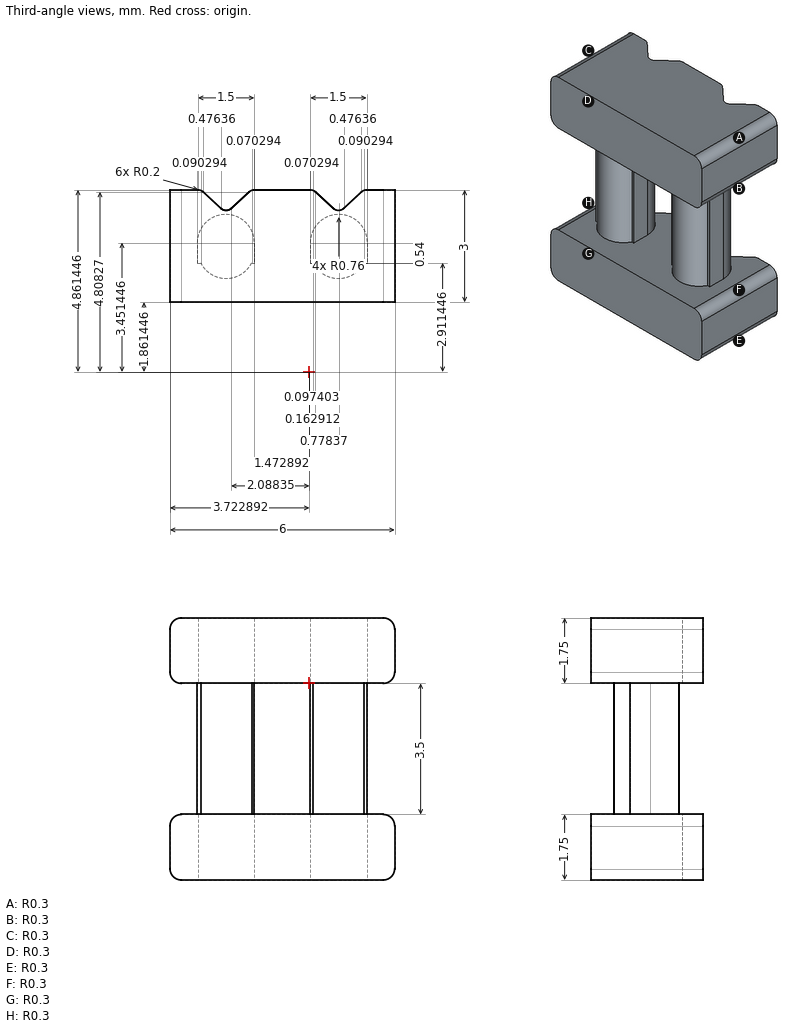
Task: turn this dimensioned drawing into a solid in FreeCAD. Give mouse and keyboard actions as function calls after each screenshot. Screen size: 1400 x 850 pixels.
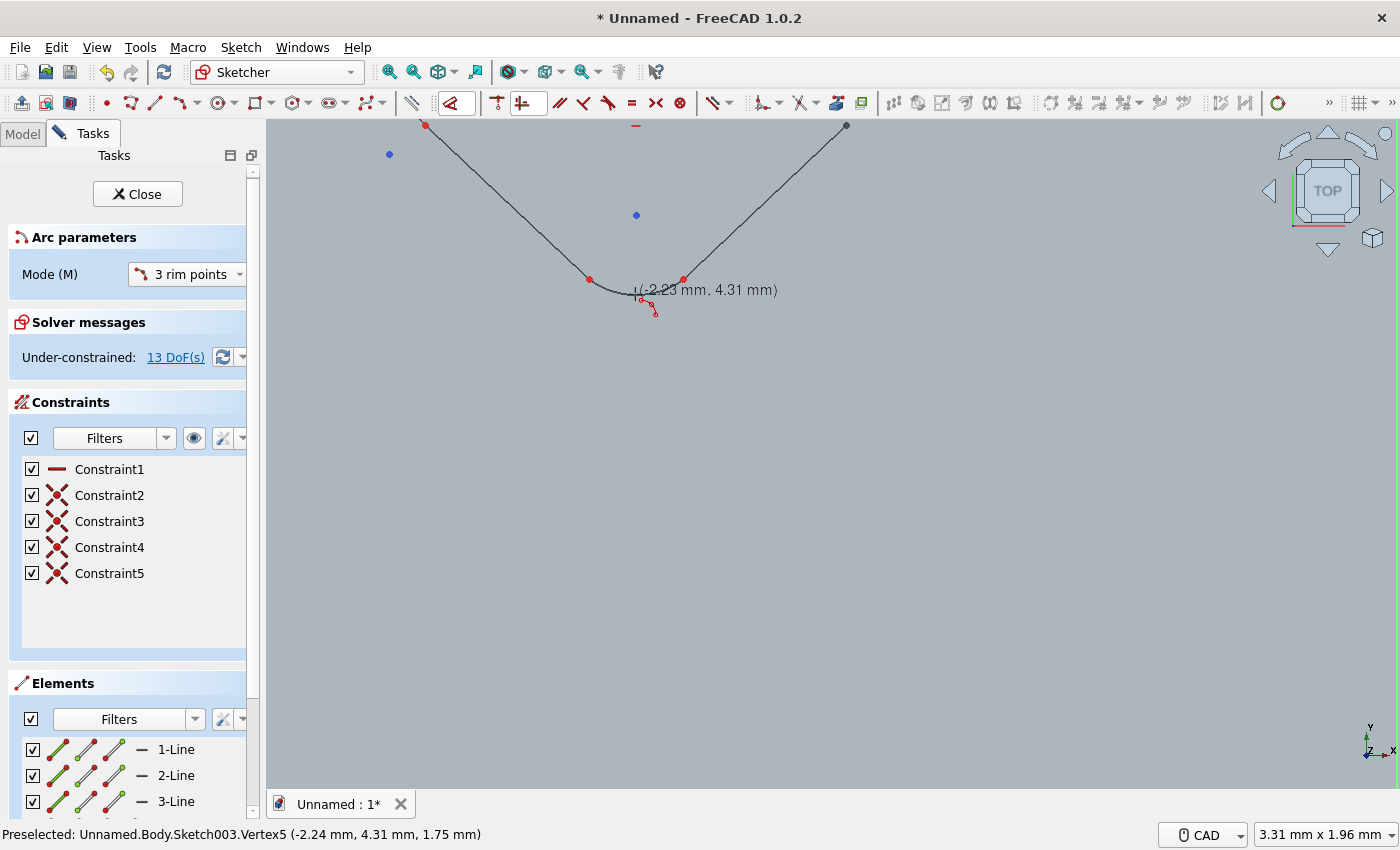
scroll(639, 296, down, 7)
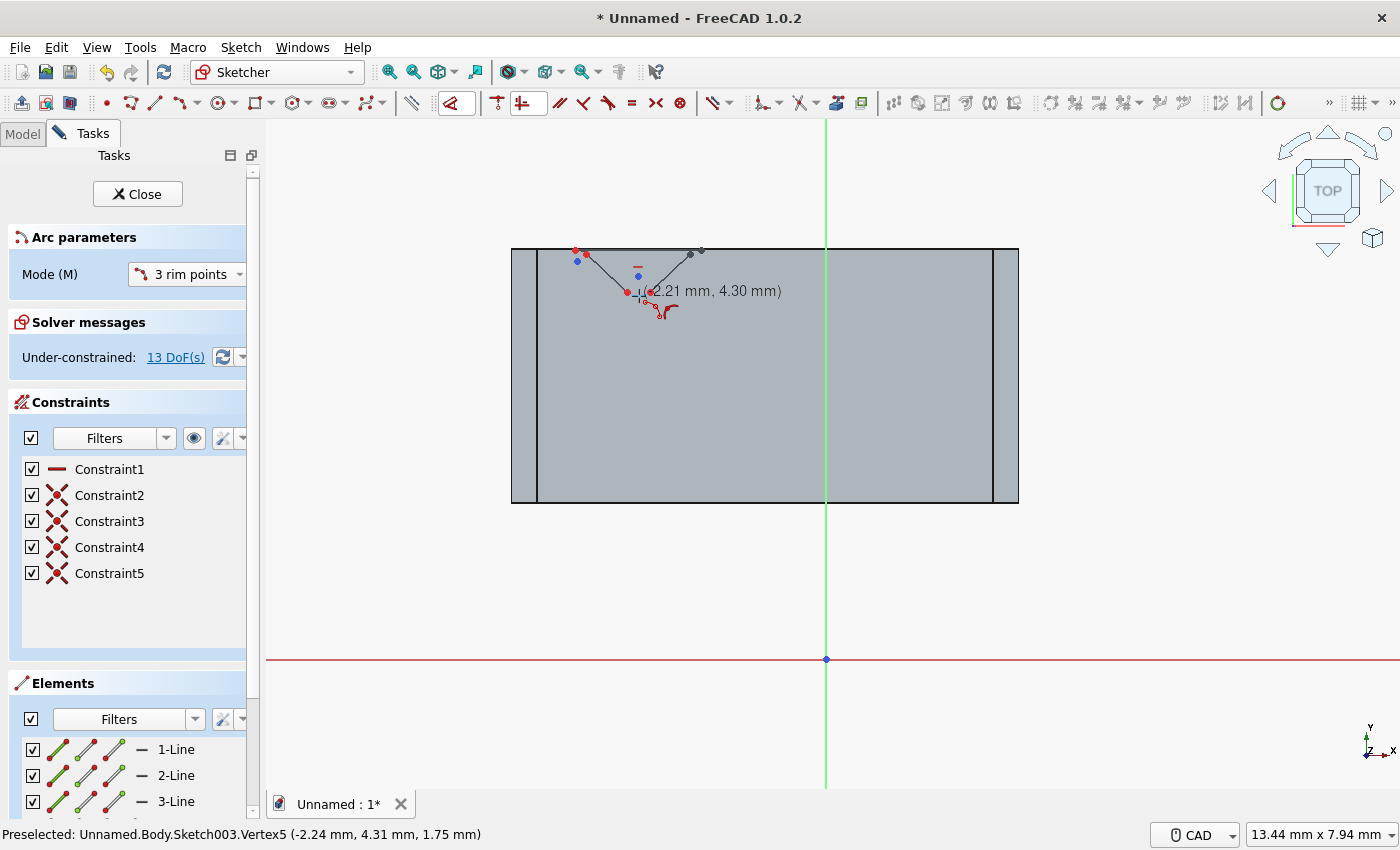
scroll(690, 254, up, 7)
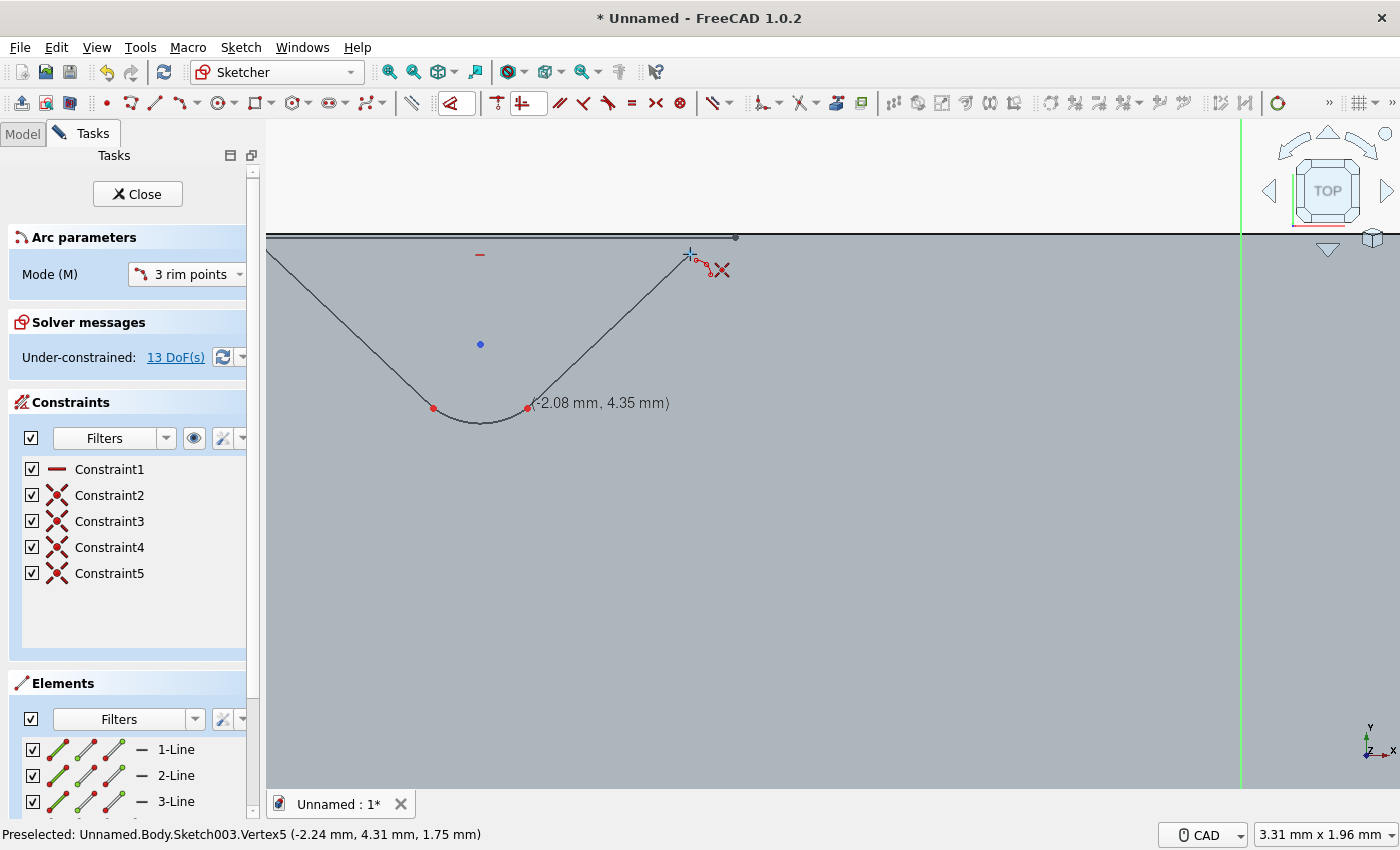
click(690, 254)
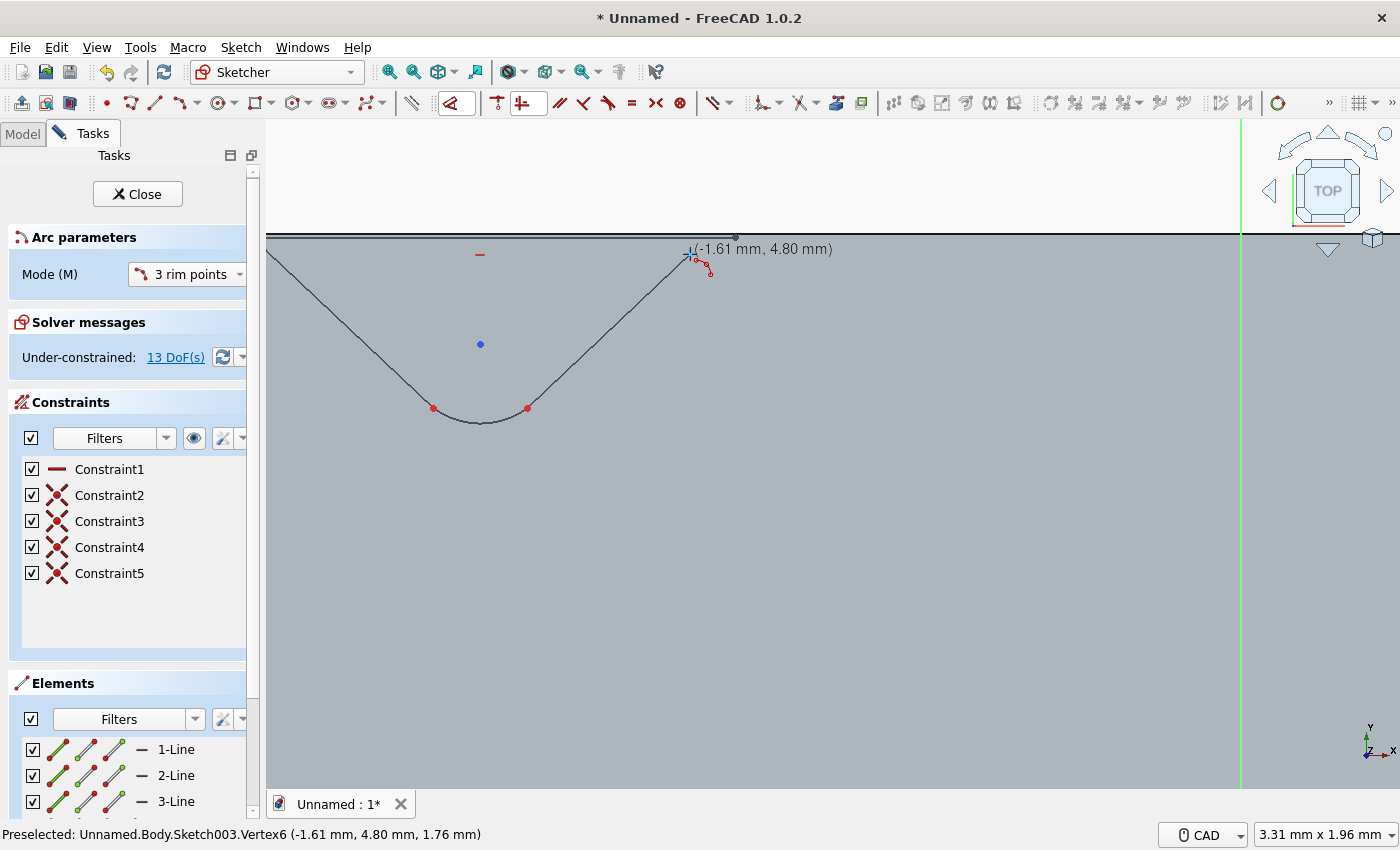
scroll(690, 254, down, 7)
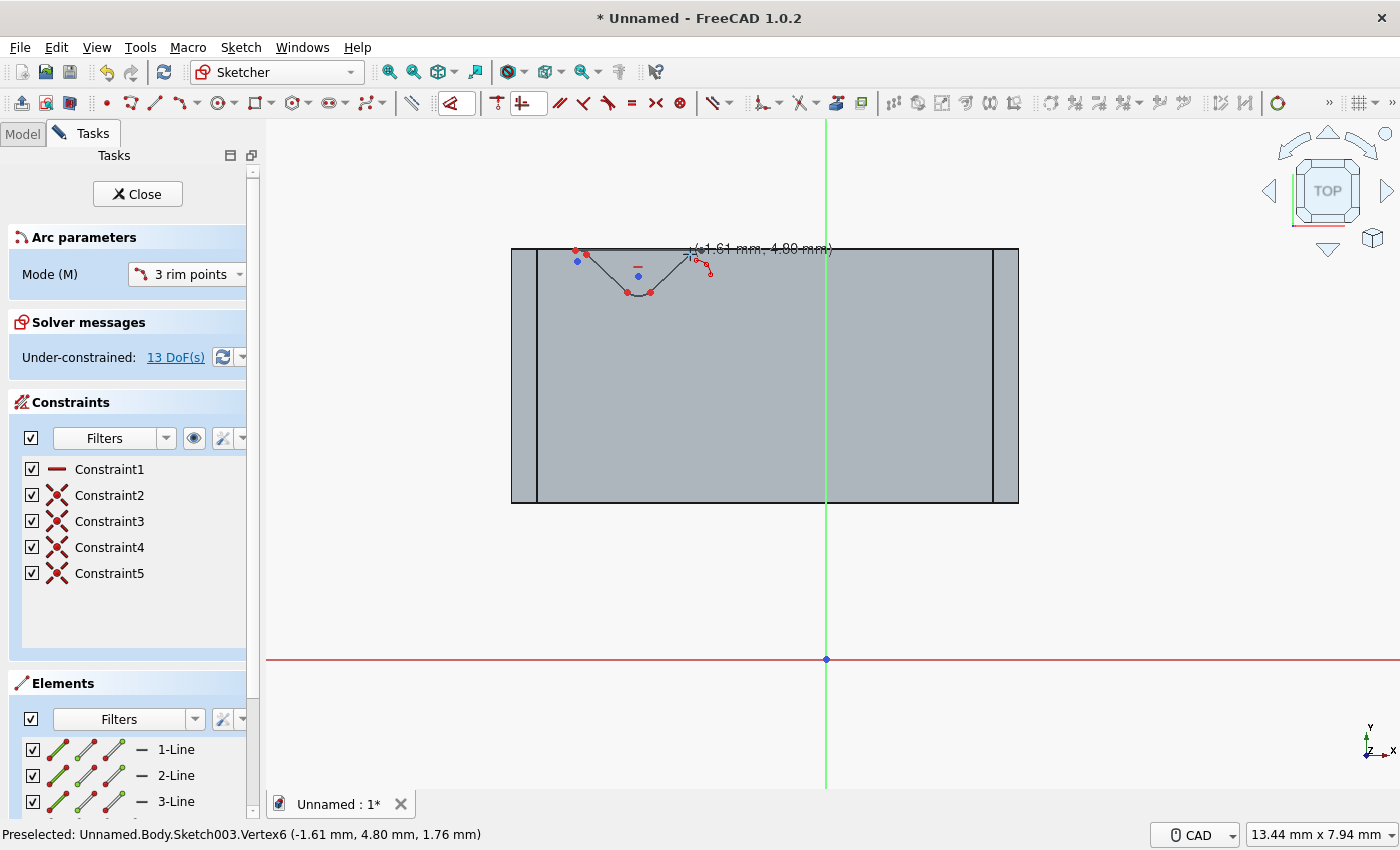
scroll(702, 249, up, 2)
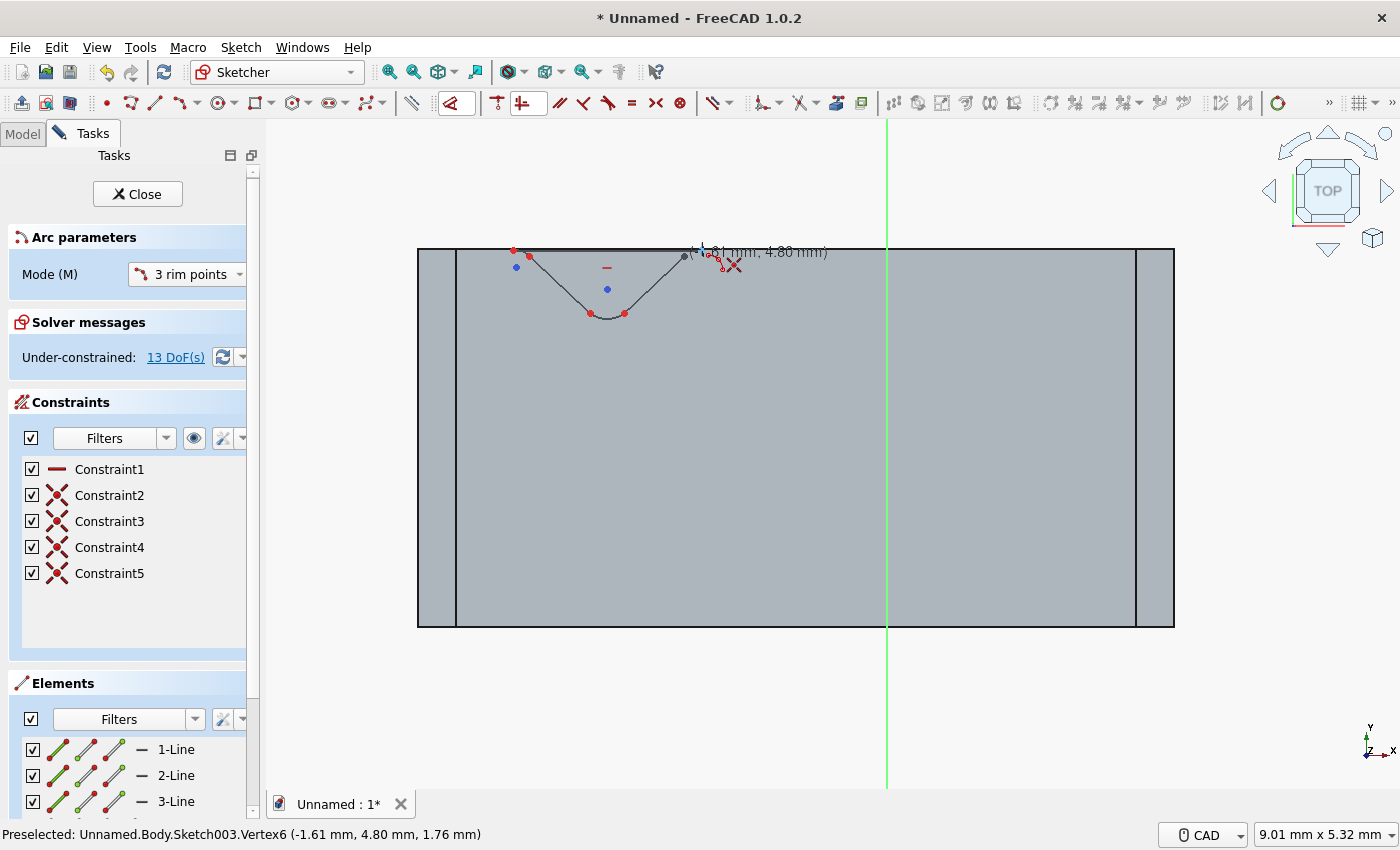
click(701, 251)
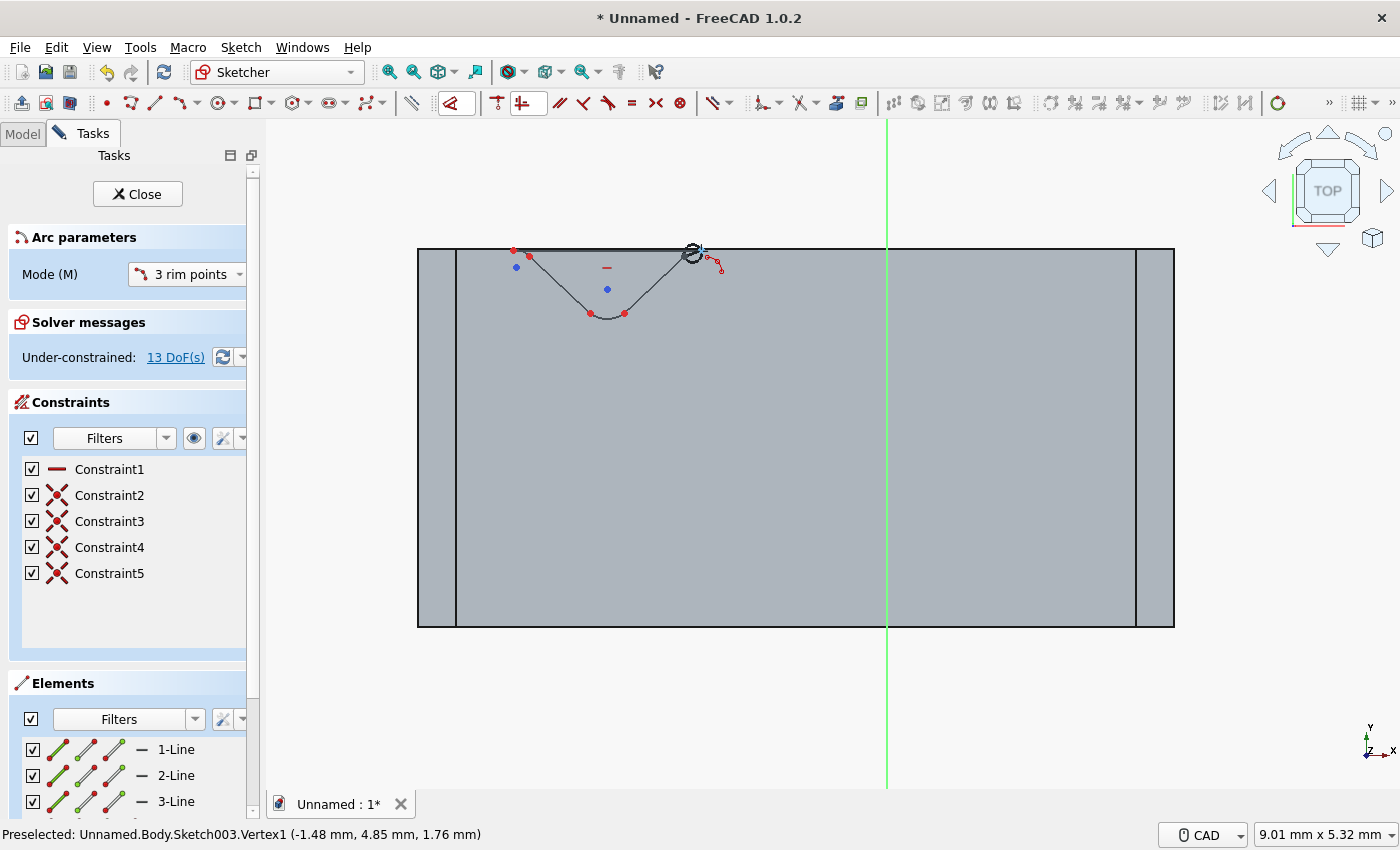
scroll(692, 251, up, 12)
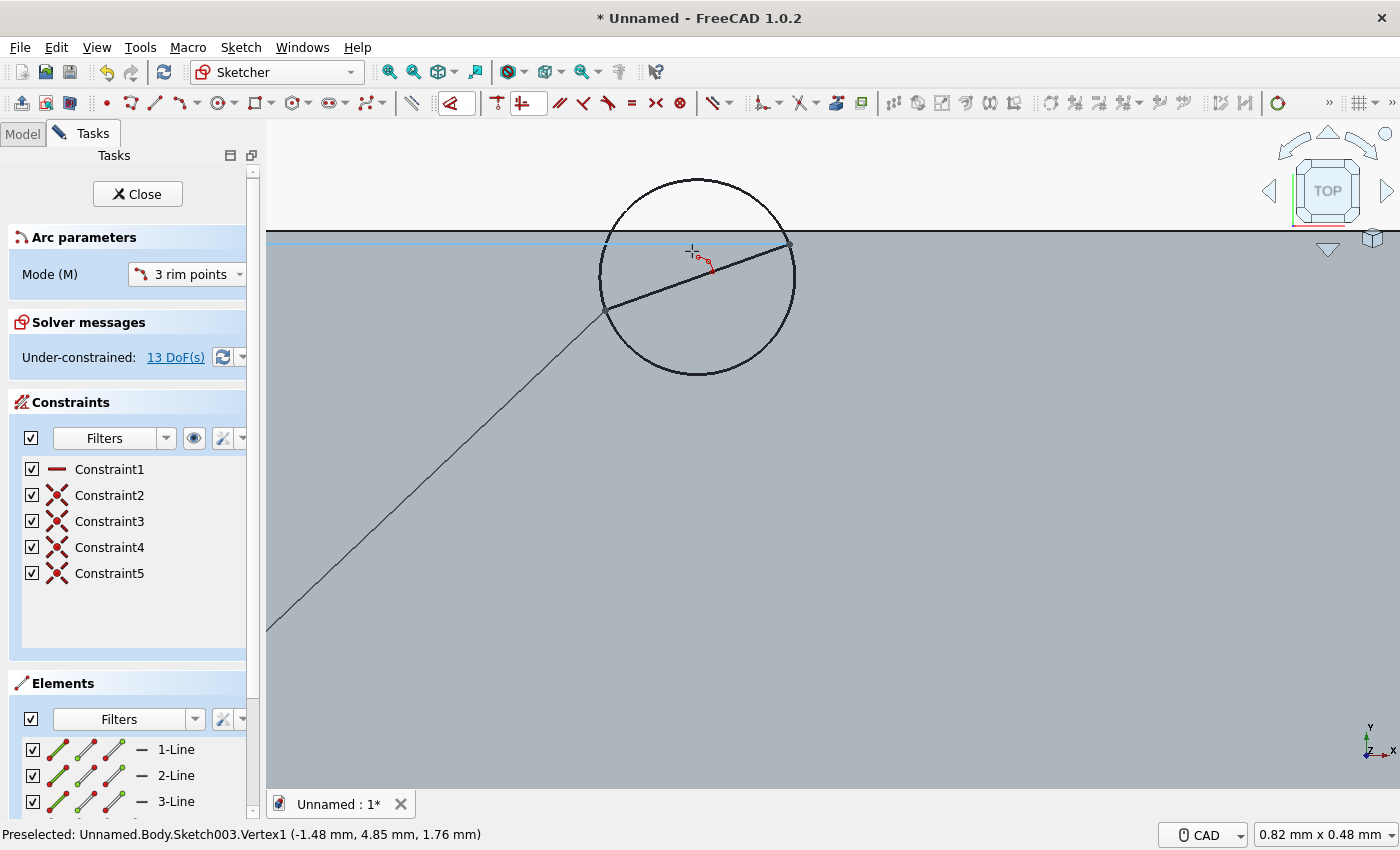
click(691, 250)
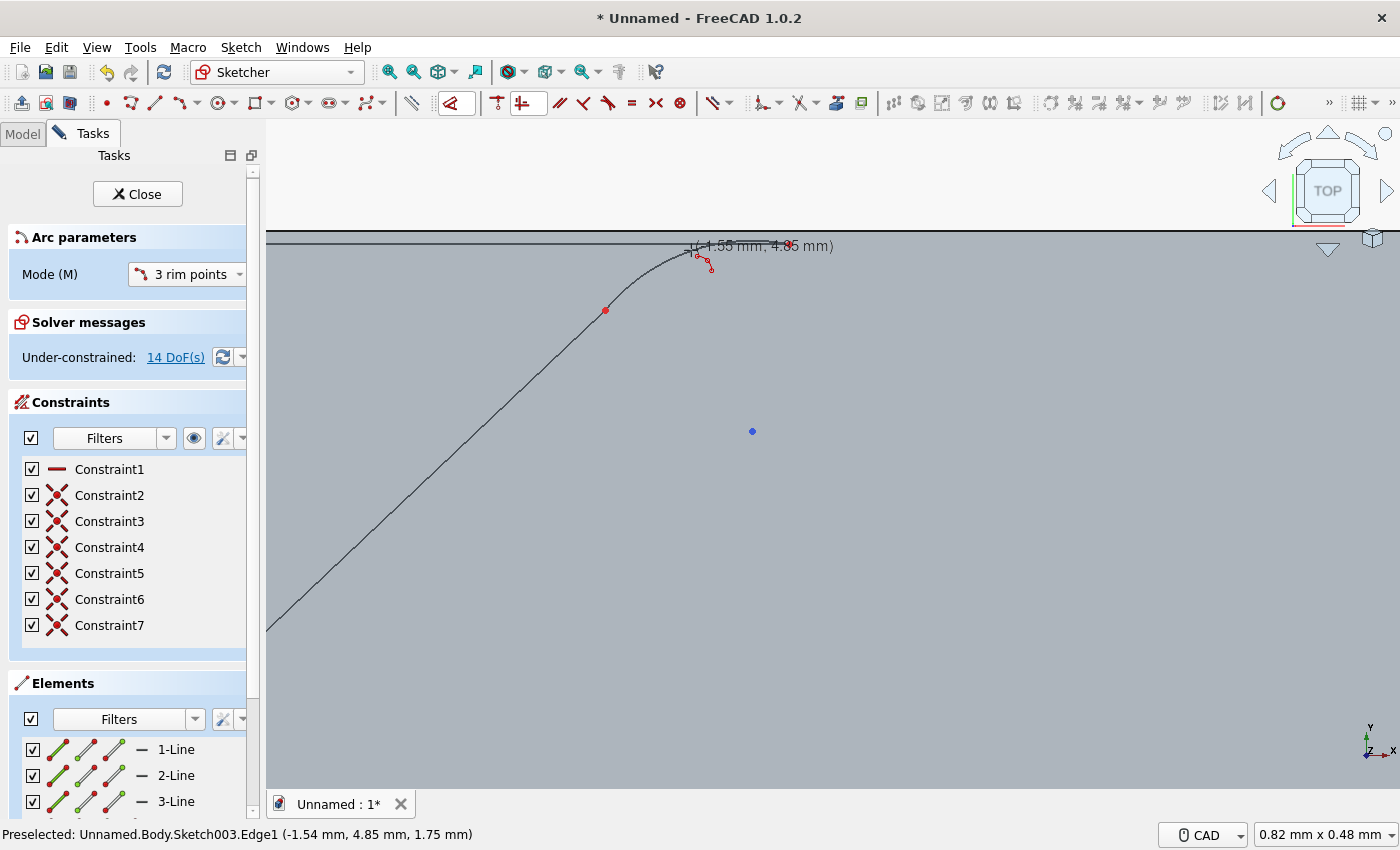
key(g)
key(l)